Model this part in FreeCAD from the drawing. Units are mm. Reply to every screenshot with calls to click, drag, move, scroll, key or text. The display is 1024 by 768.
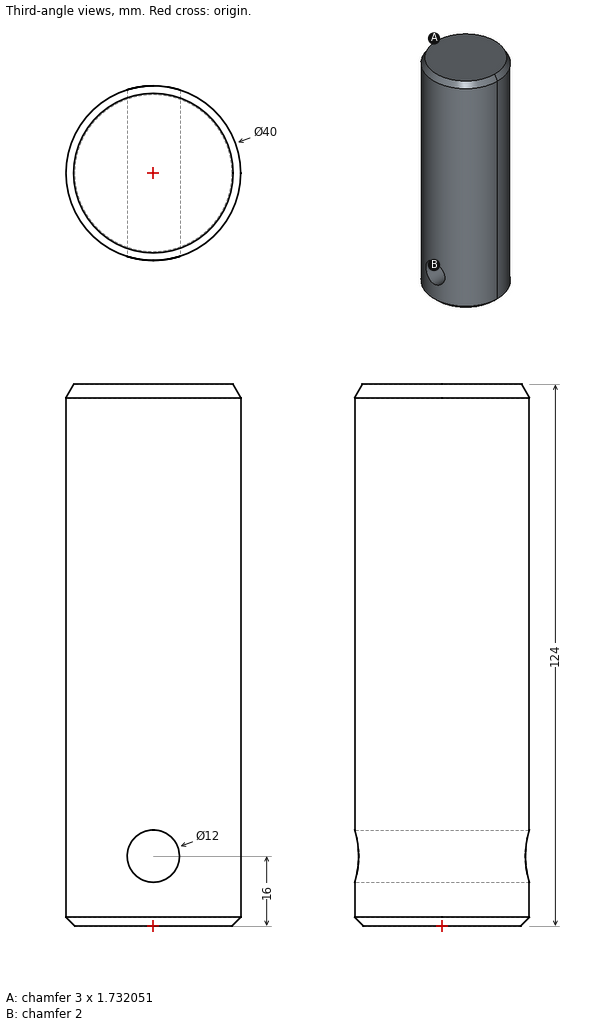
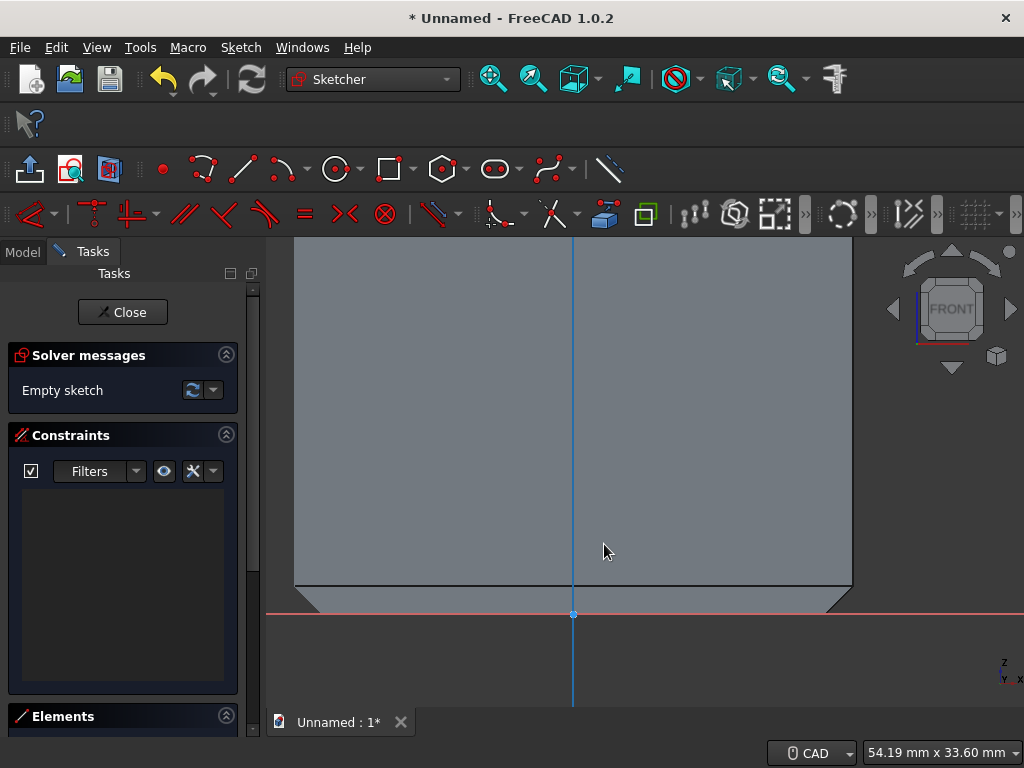
click(336, 170)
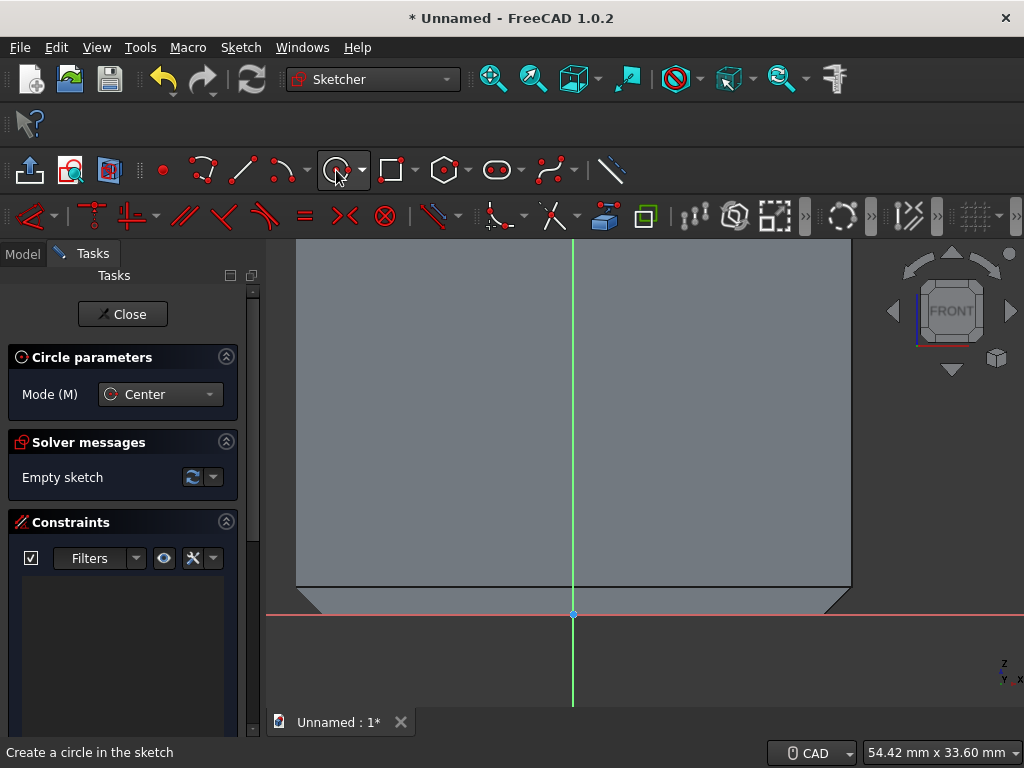
click(573, 392)
move(632, 333)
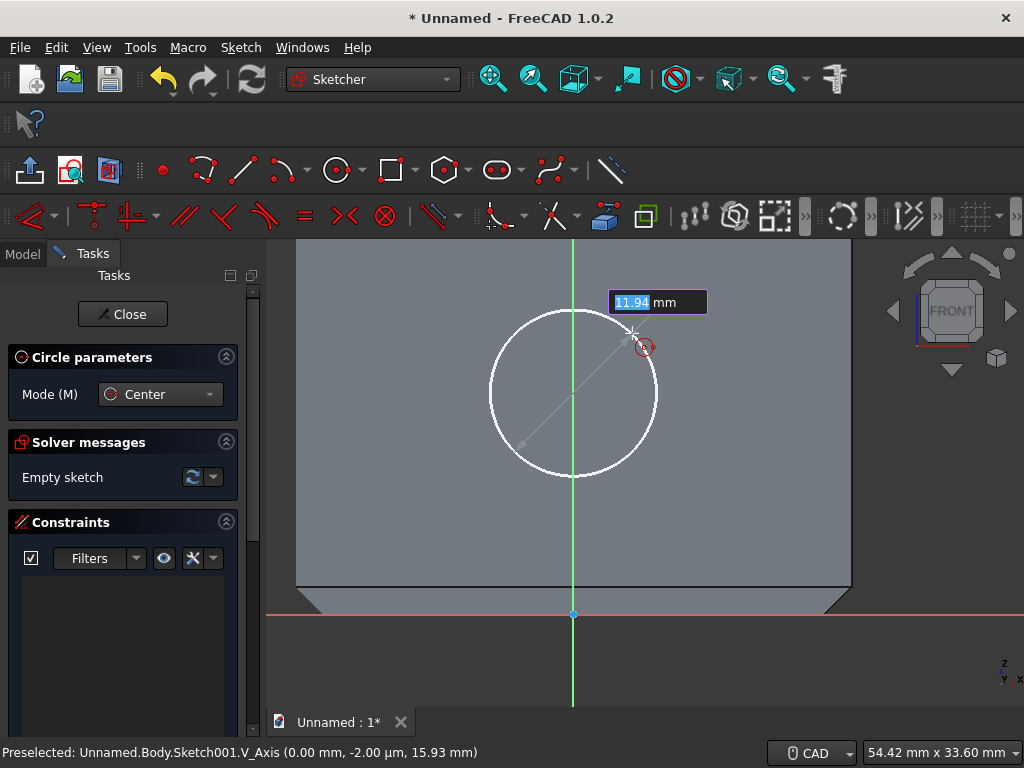
text(12)
key(Return)
key(Escape)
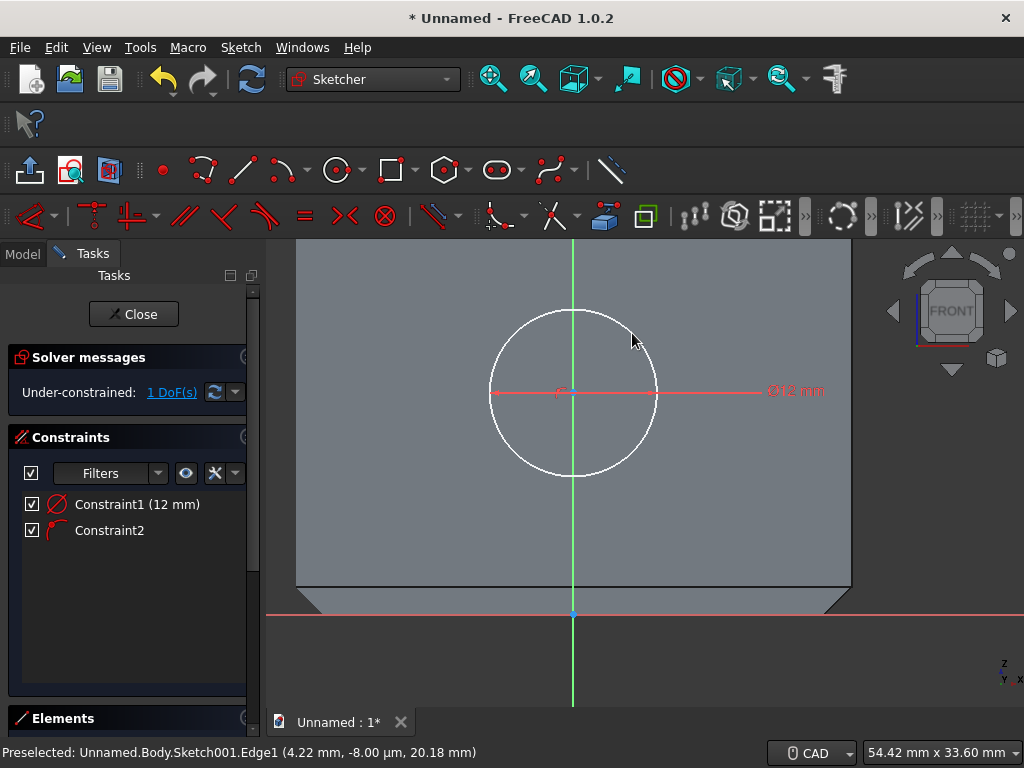
click(573, 393)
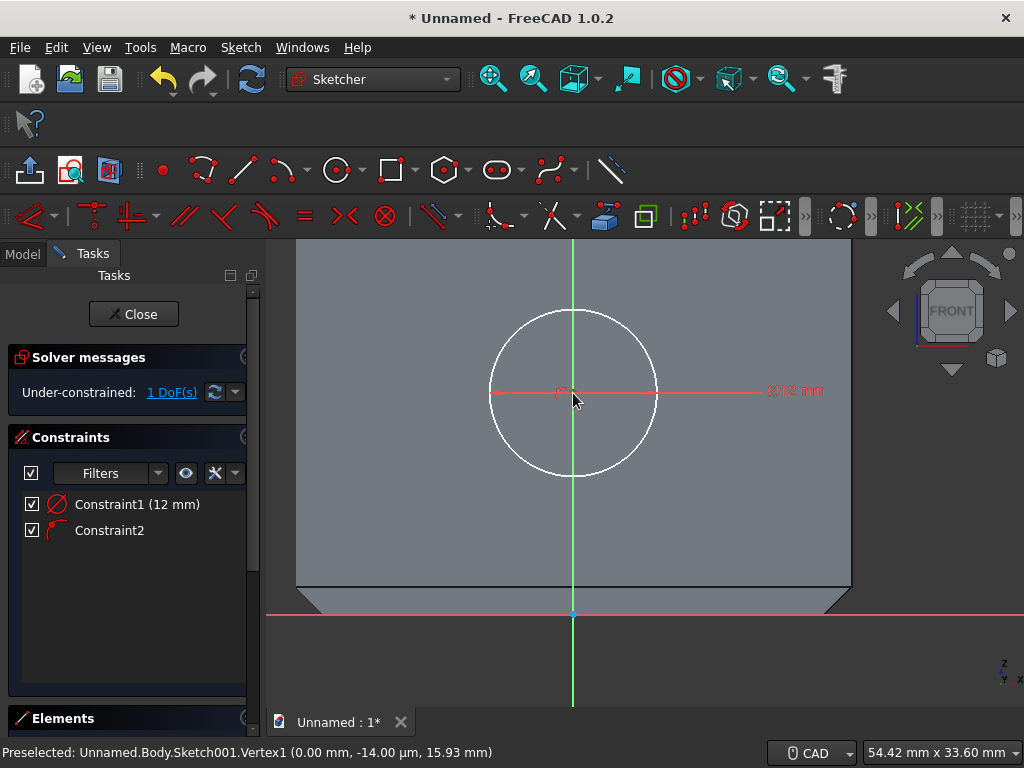
click(56, 216)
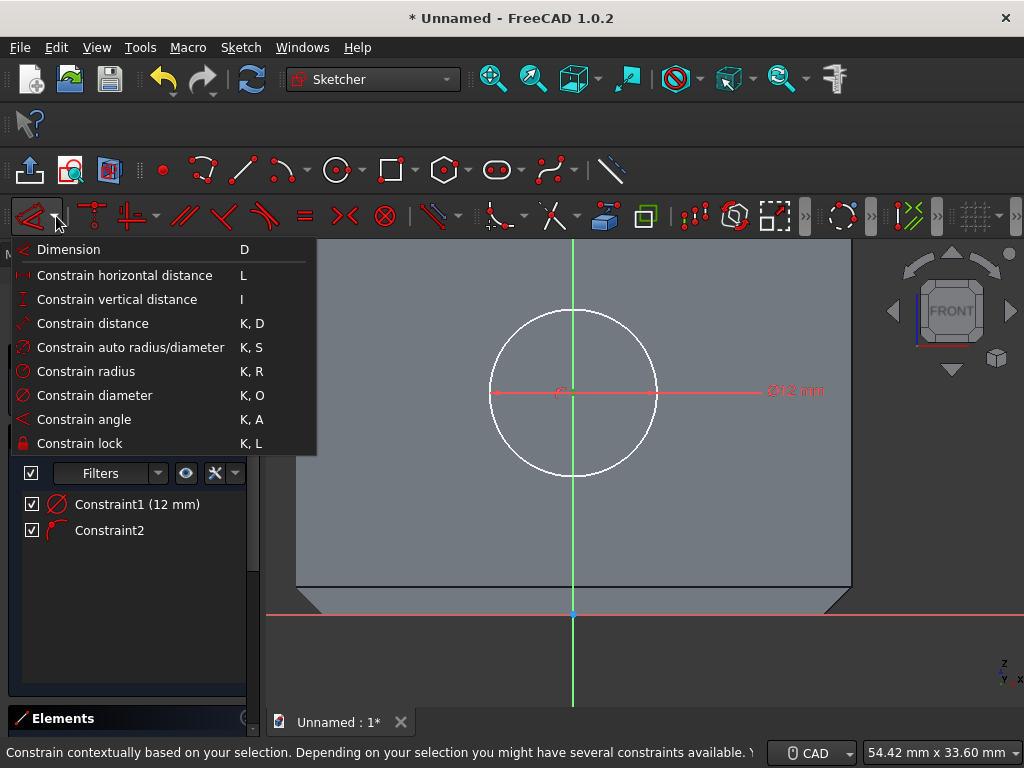
click(164, 299)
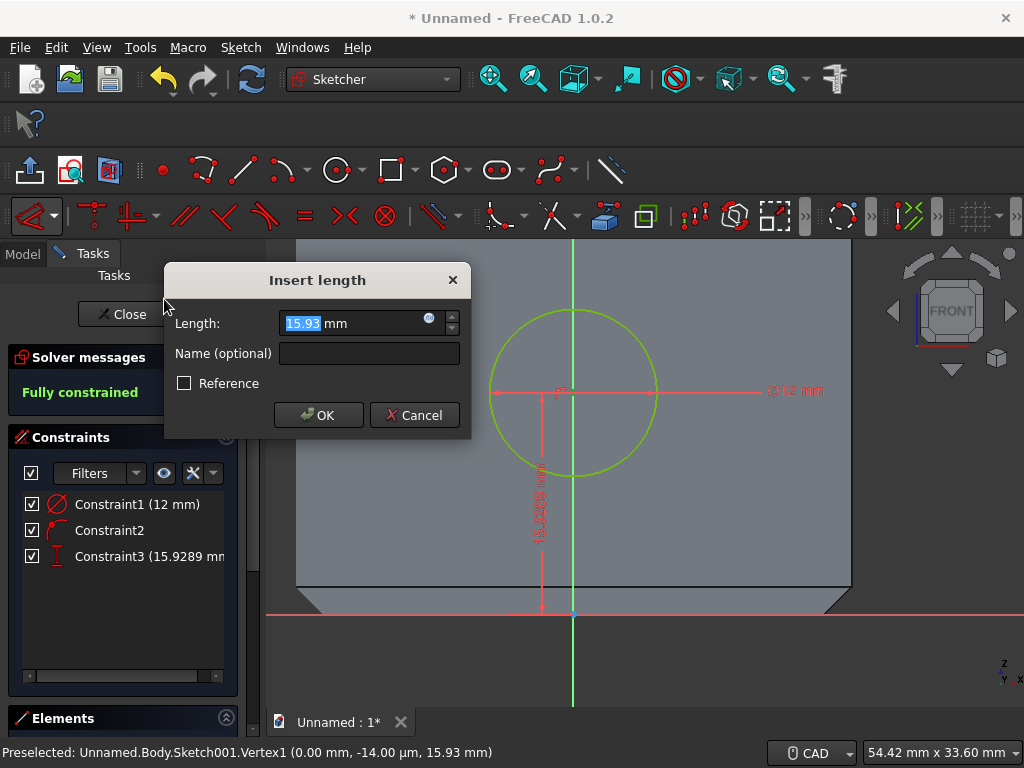
text(16)
key(Return)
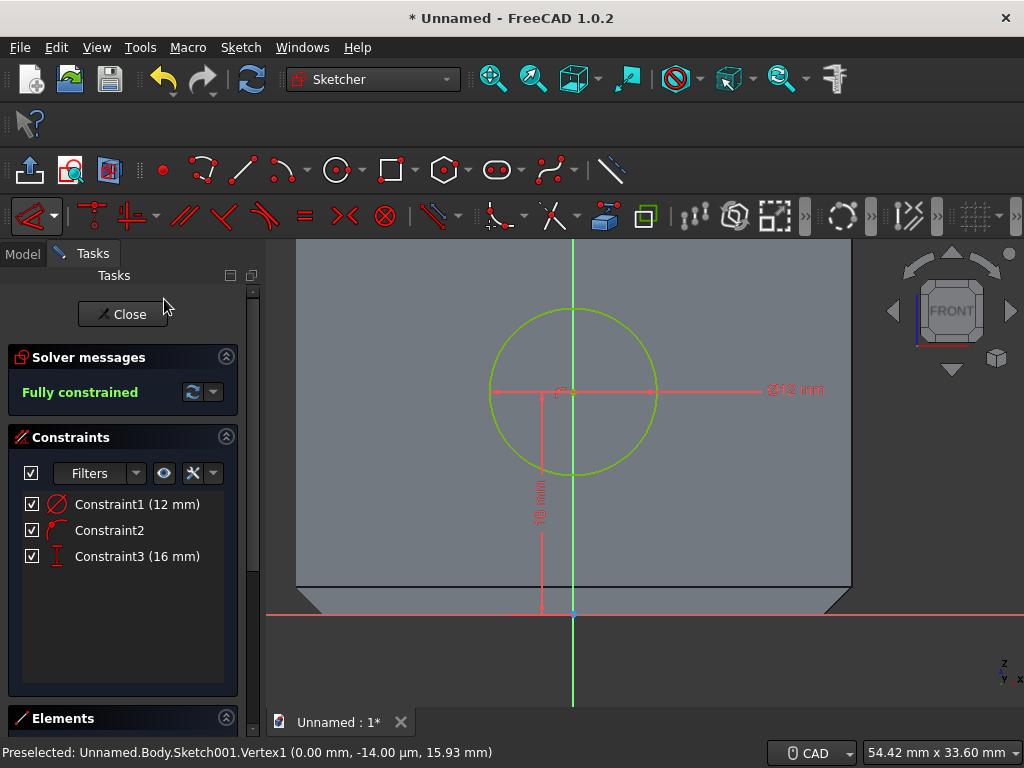
click(123, 314)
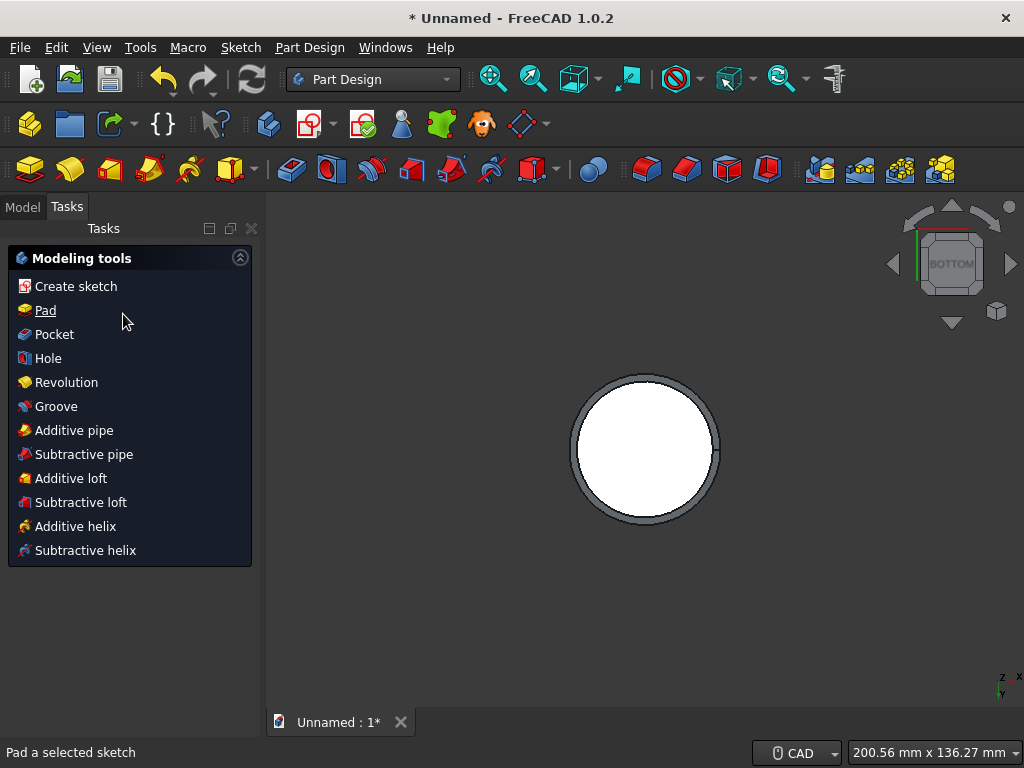
click(292, 170)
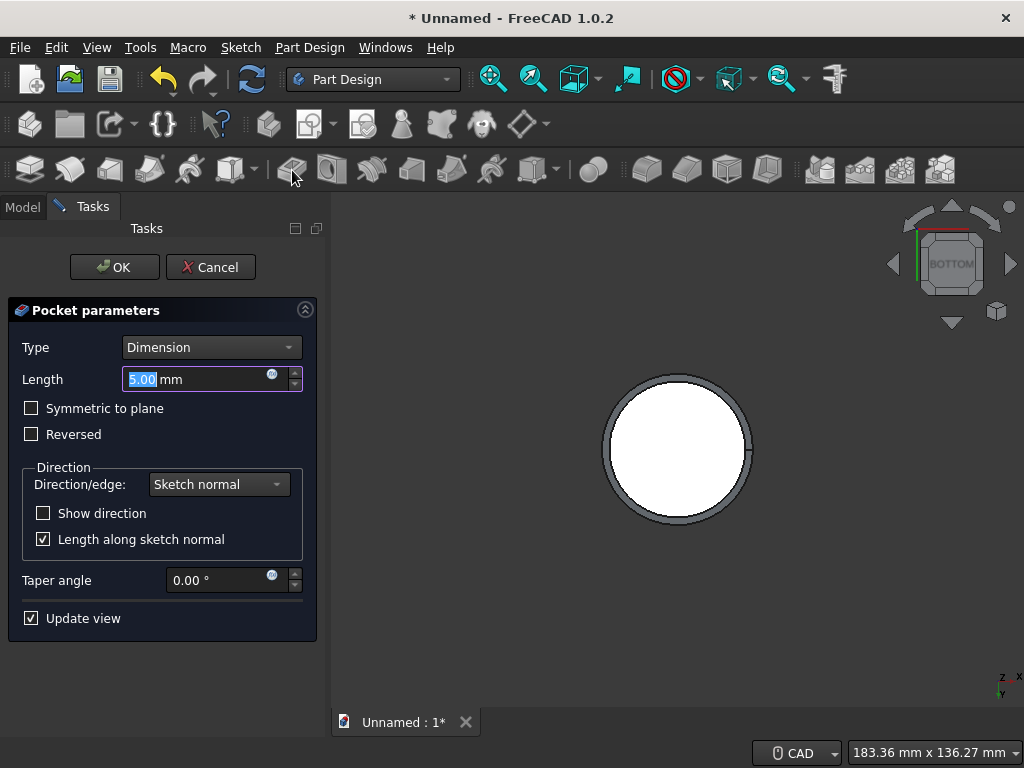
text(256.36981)
key(Tab)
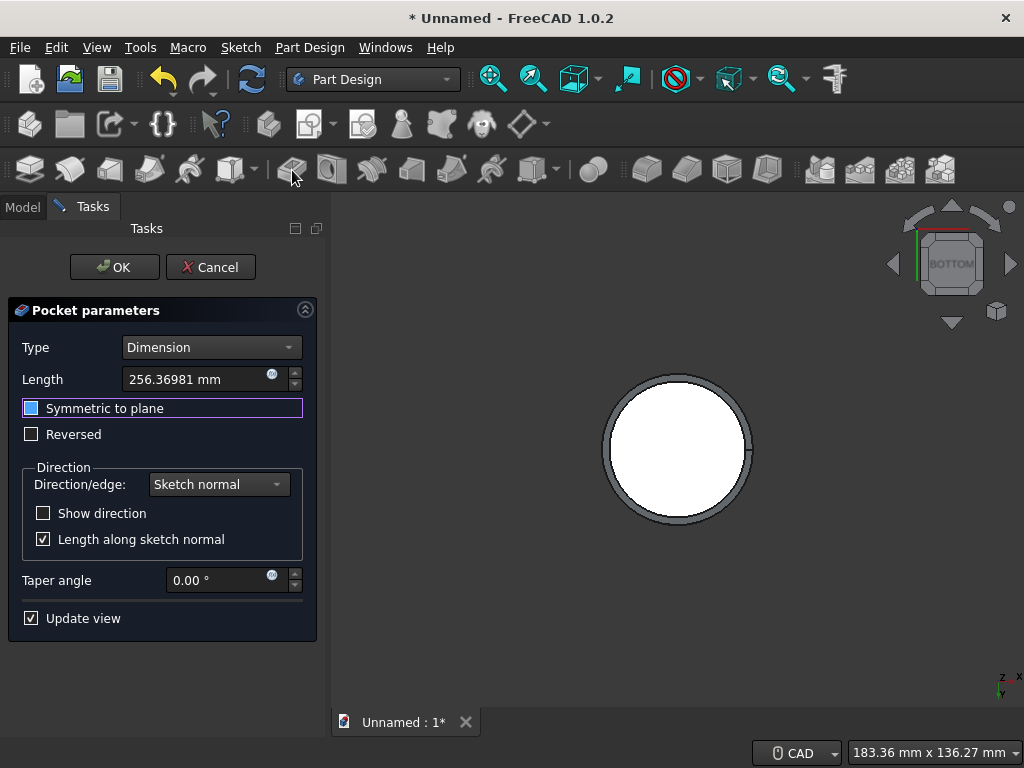
click(30, 408)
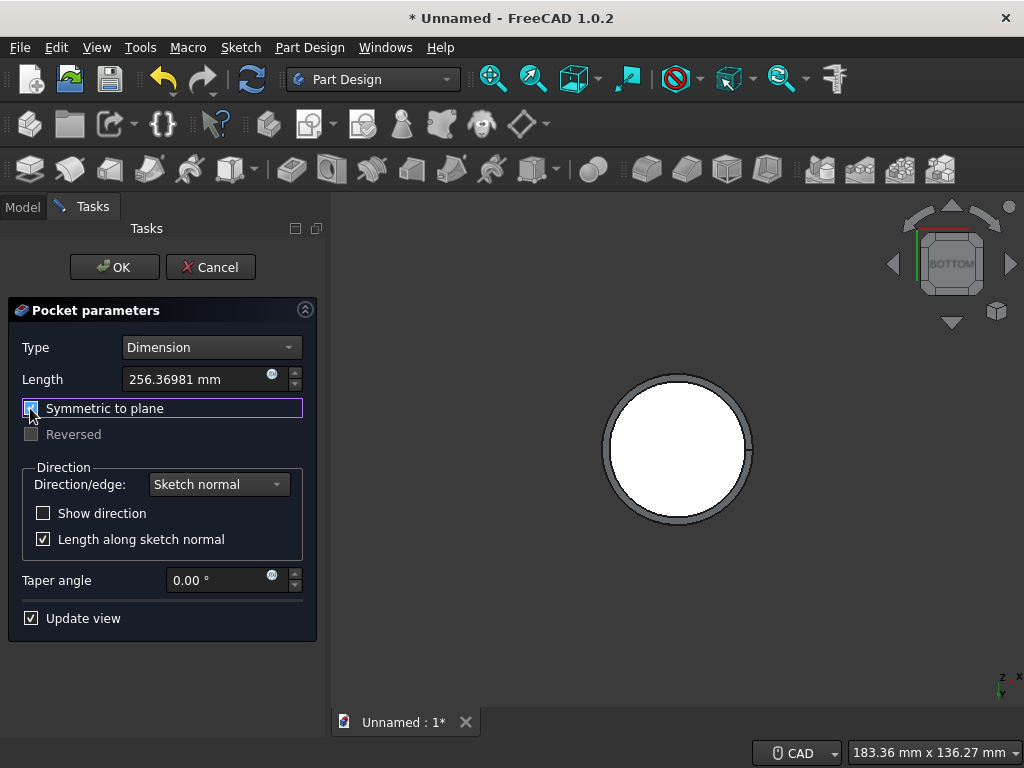
click(115, 267)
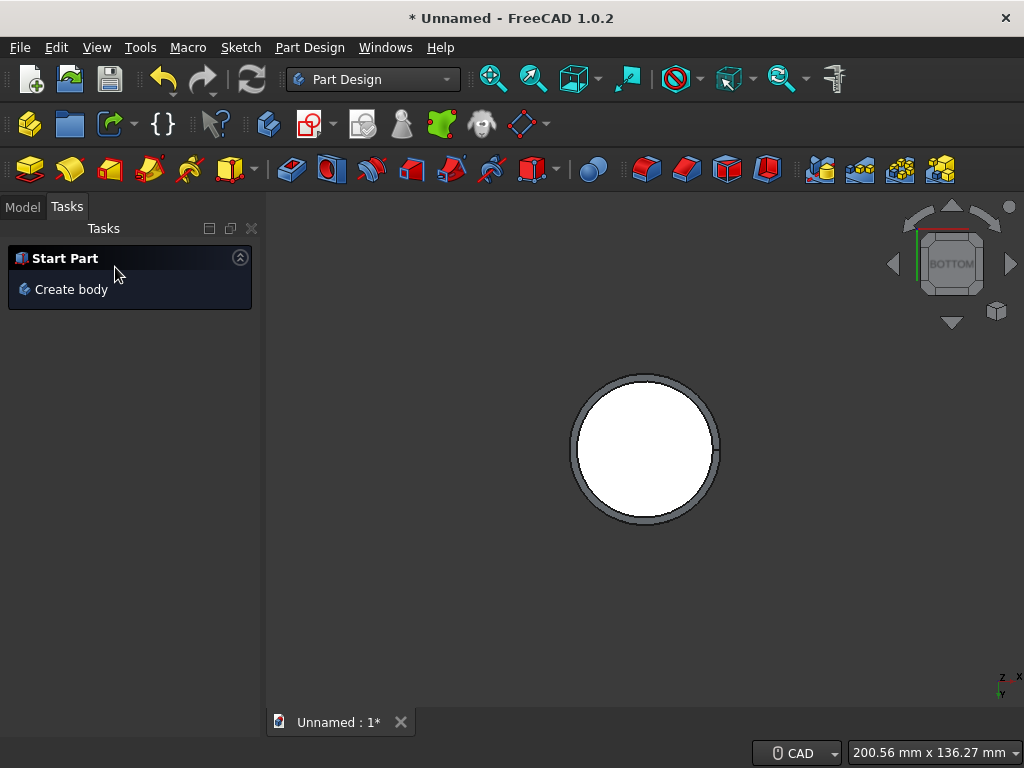
key(0)